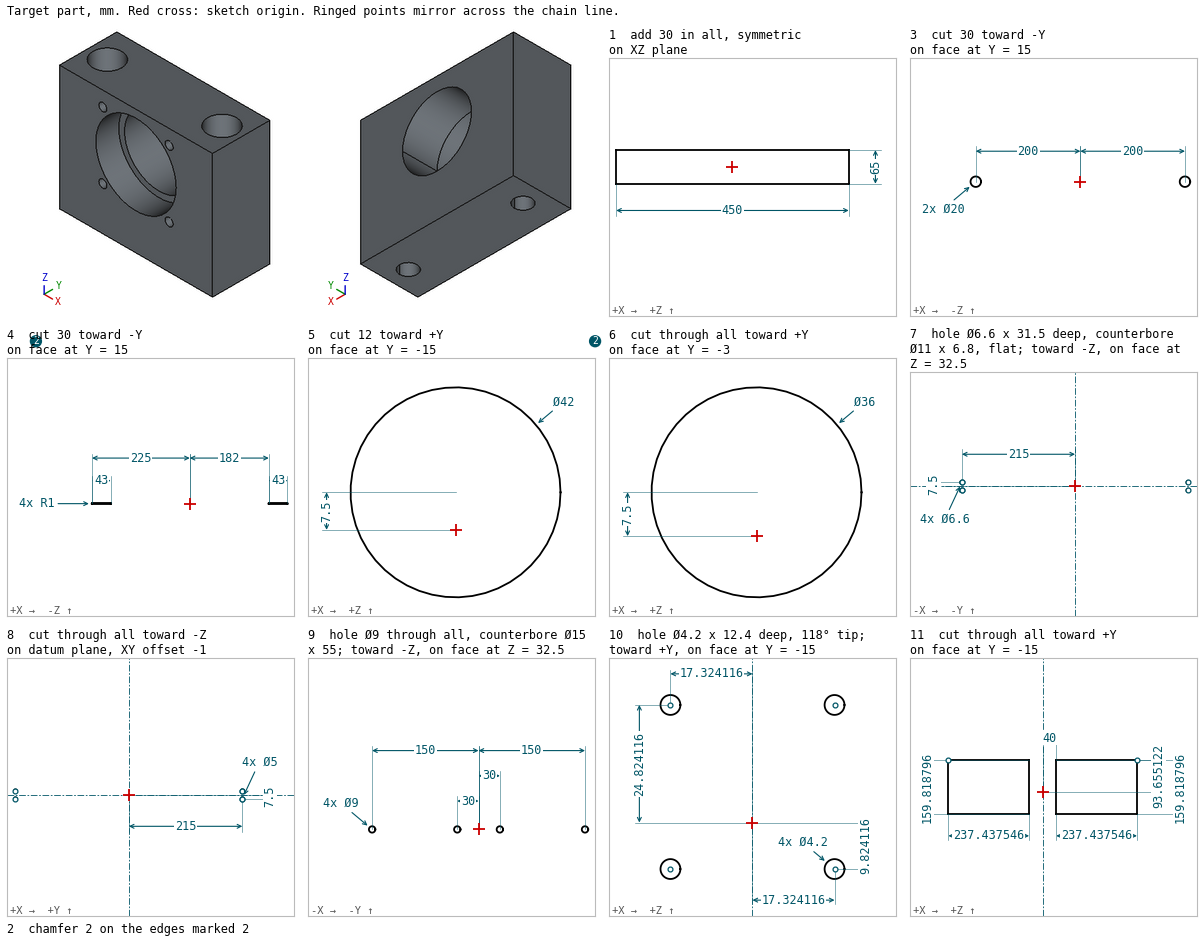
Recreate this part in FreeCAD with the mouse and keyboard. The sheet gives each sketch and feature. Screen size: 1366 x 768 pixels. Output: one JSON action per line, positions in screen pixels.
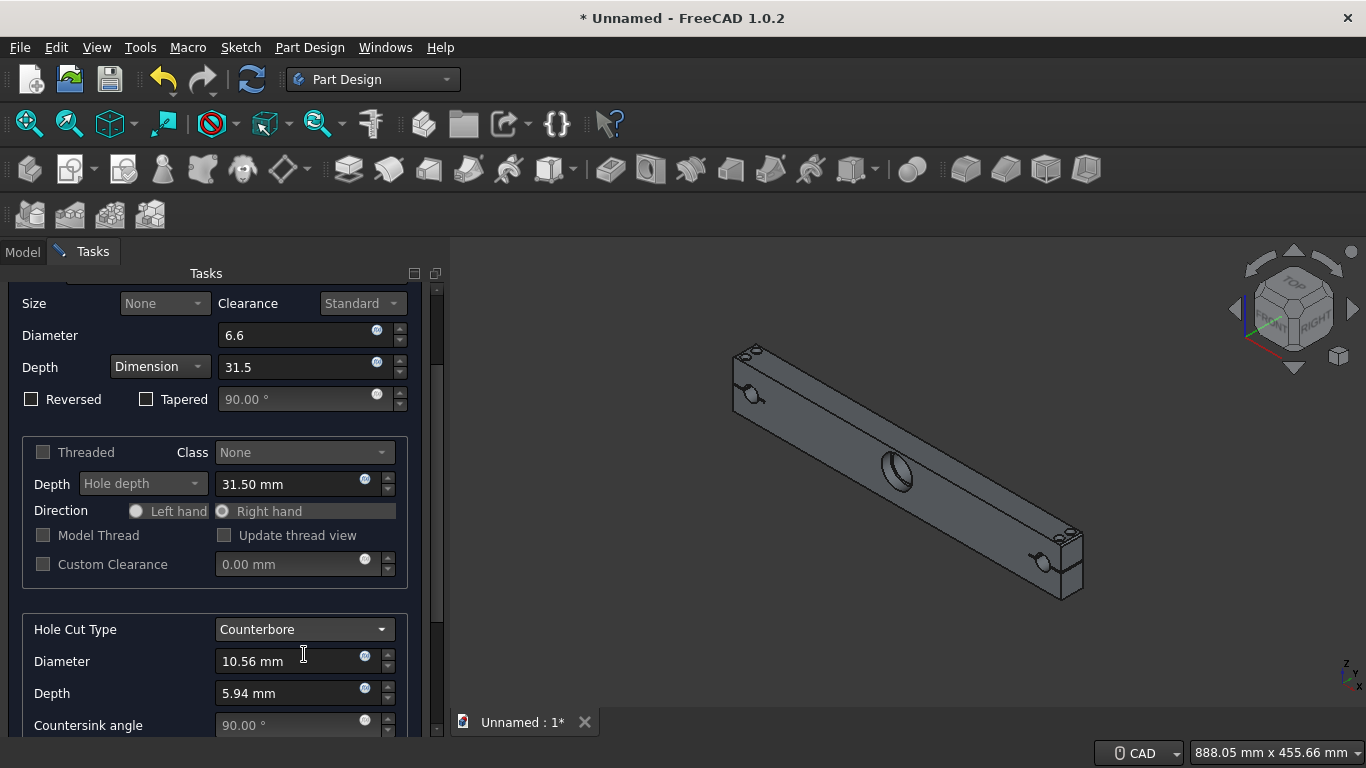
{"action": "triple_click", "coordinate": [298, 661]}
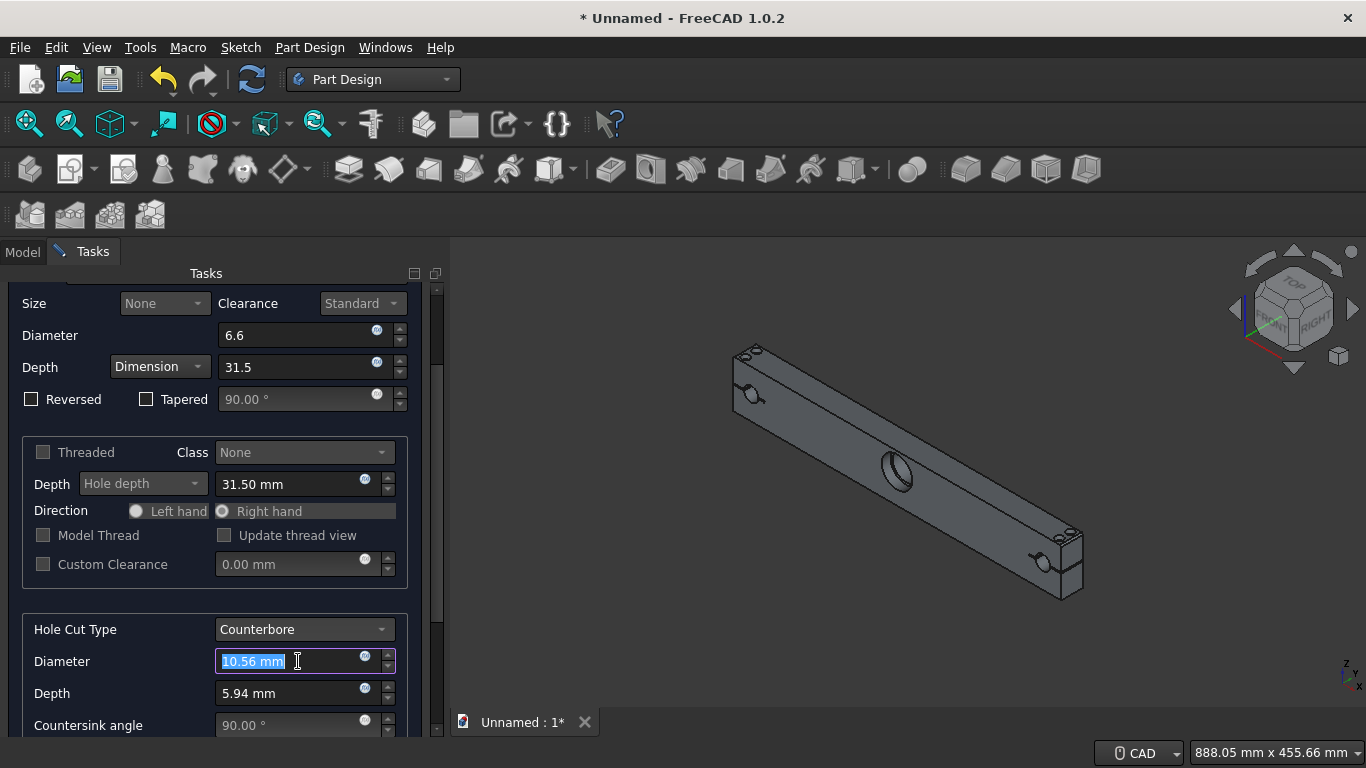
{"action": "type", "text": "11"}
{"action": "key", "text": "Tab"}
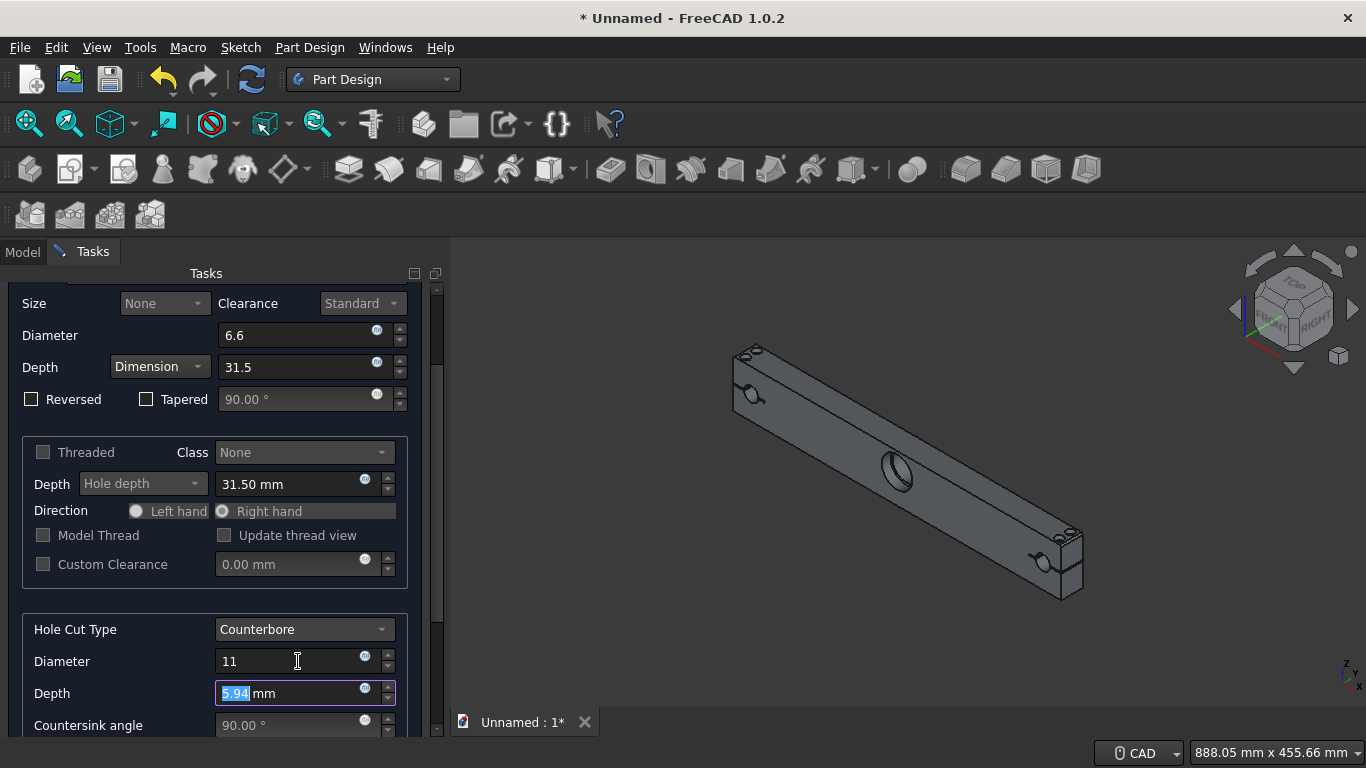
{"action": "type", "text": "6.8"}
{"action": "key", "text": "Tab"}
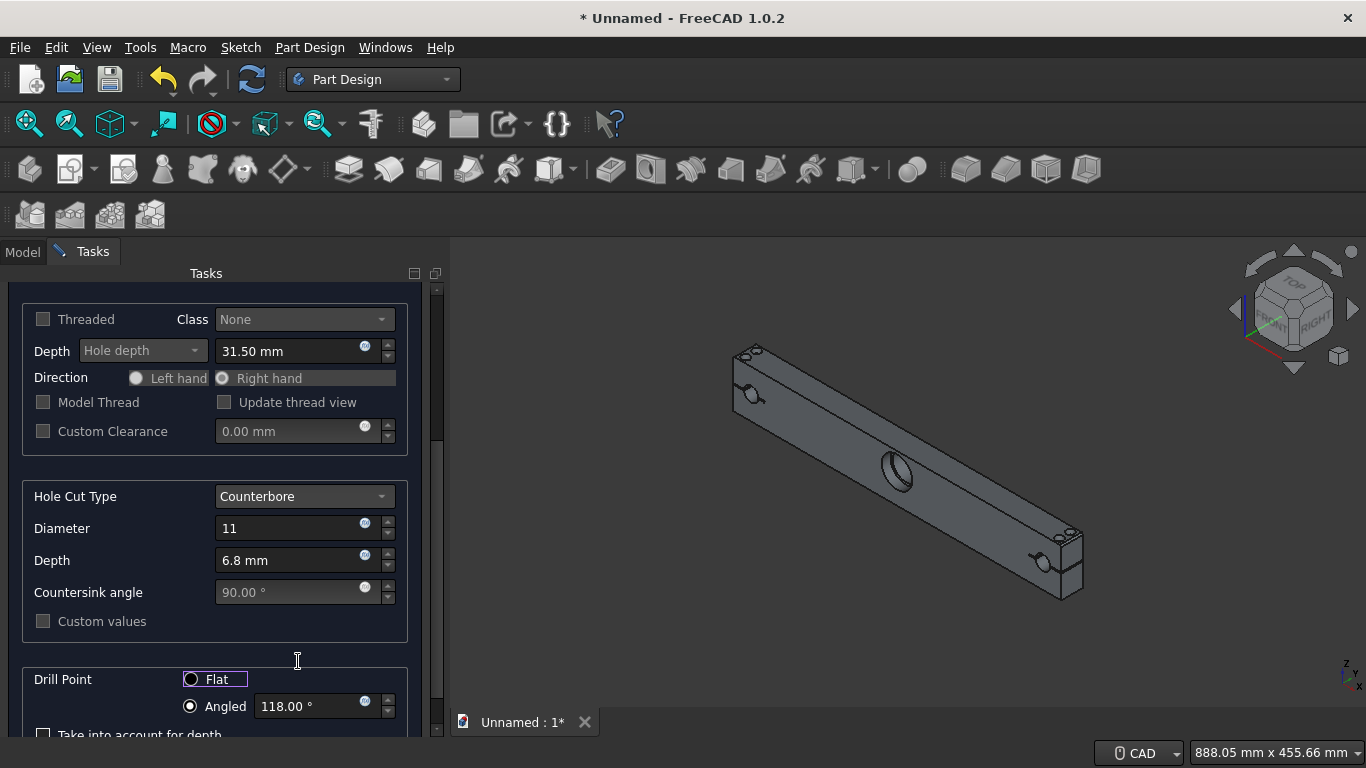
{"action": "left_click", "coordinate": [191, 679]}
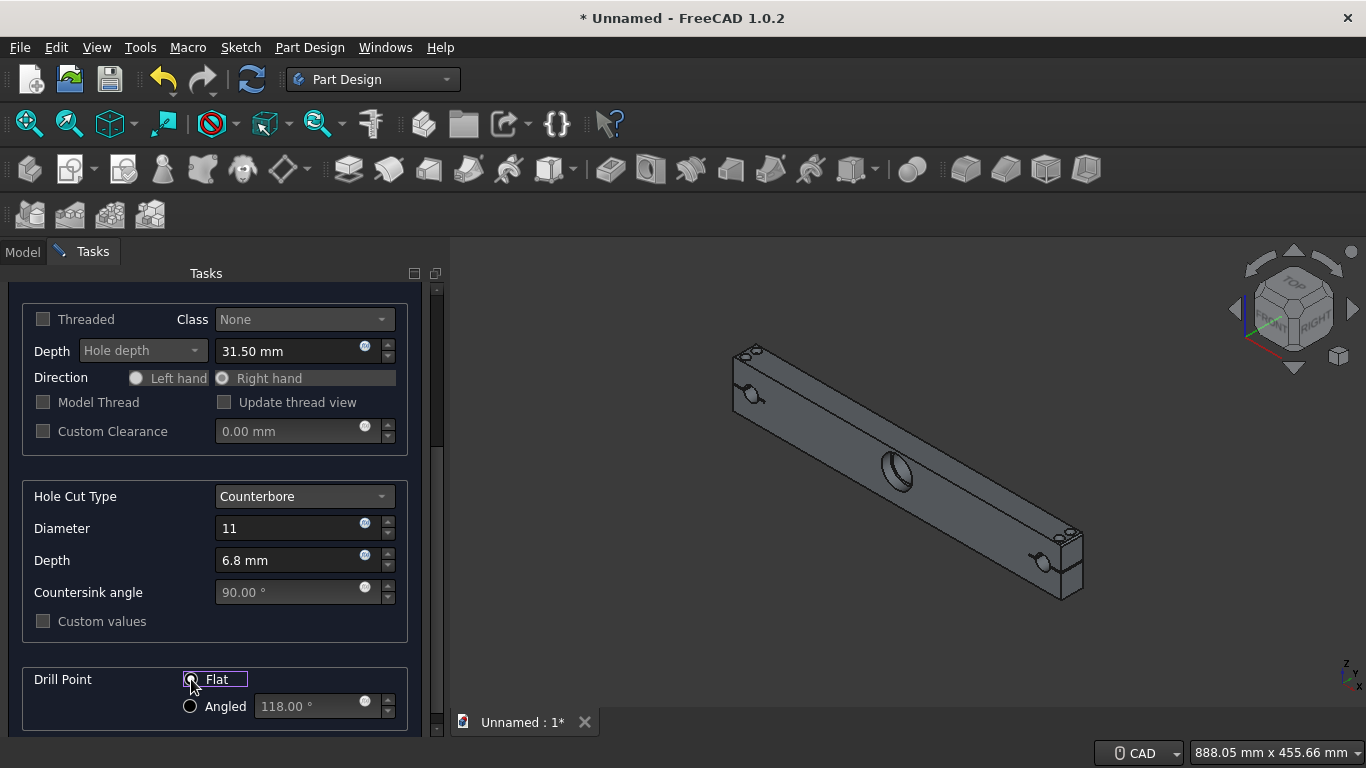
{"action": "scroll", "coordinate": [437, 510], "scroll_direction": "up", "scroll_amount": 5}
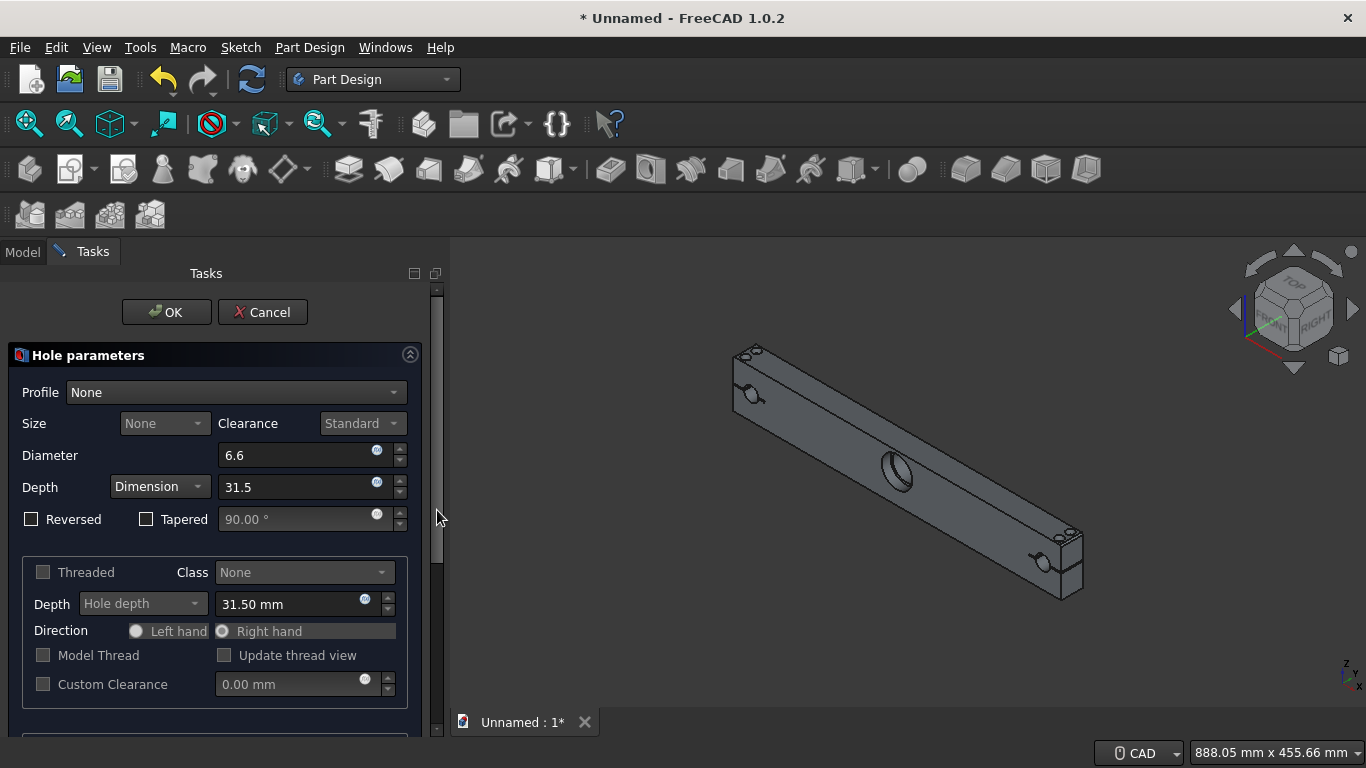
{"action": "left_click", "coordinate": [167, 312]}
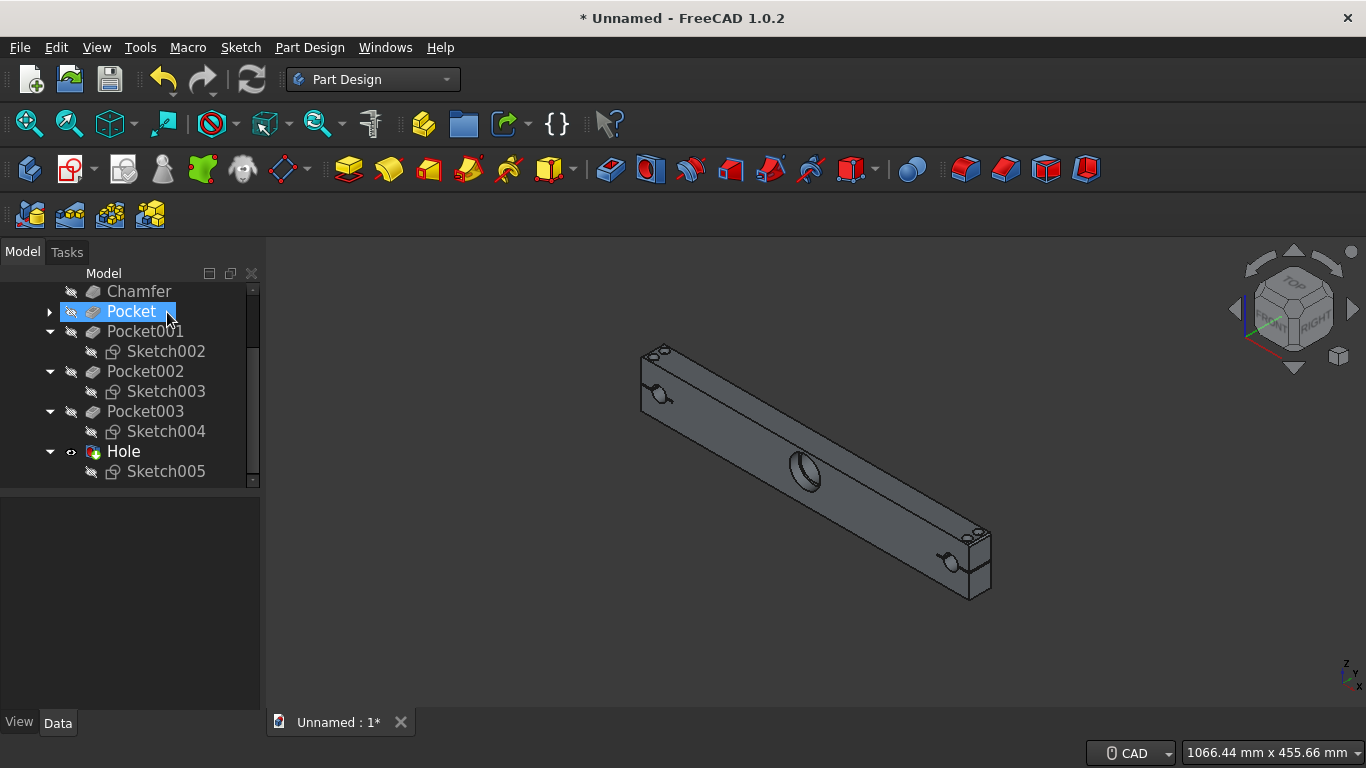
{"action": "key", "text": "2"}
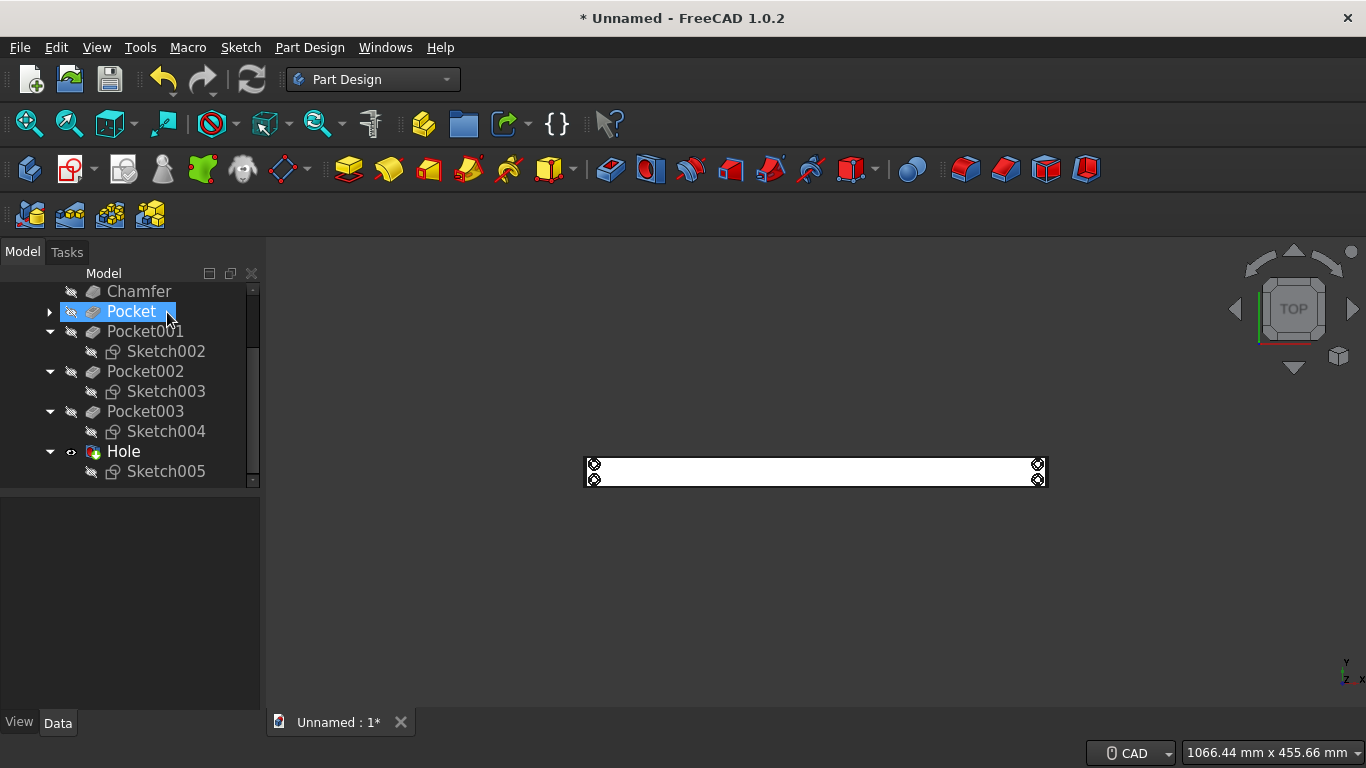
{"action": "key", "text": "v f"}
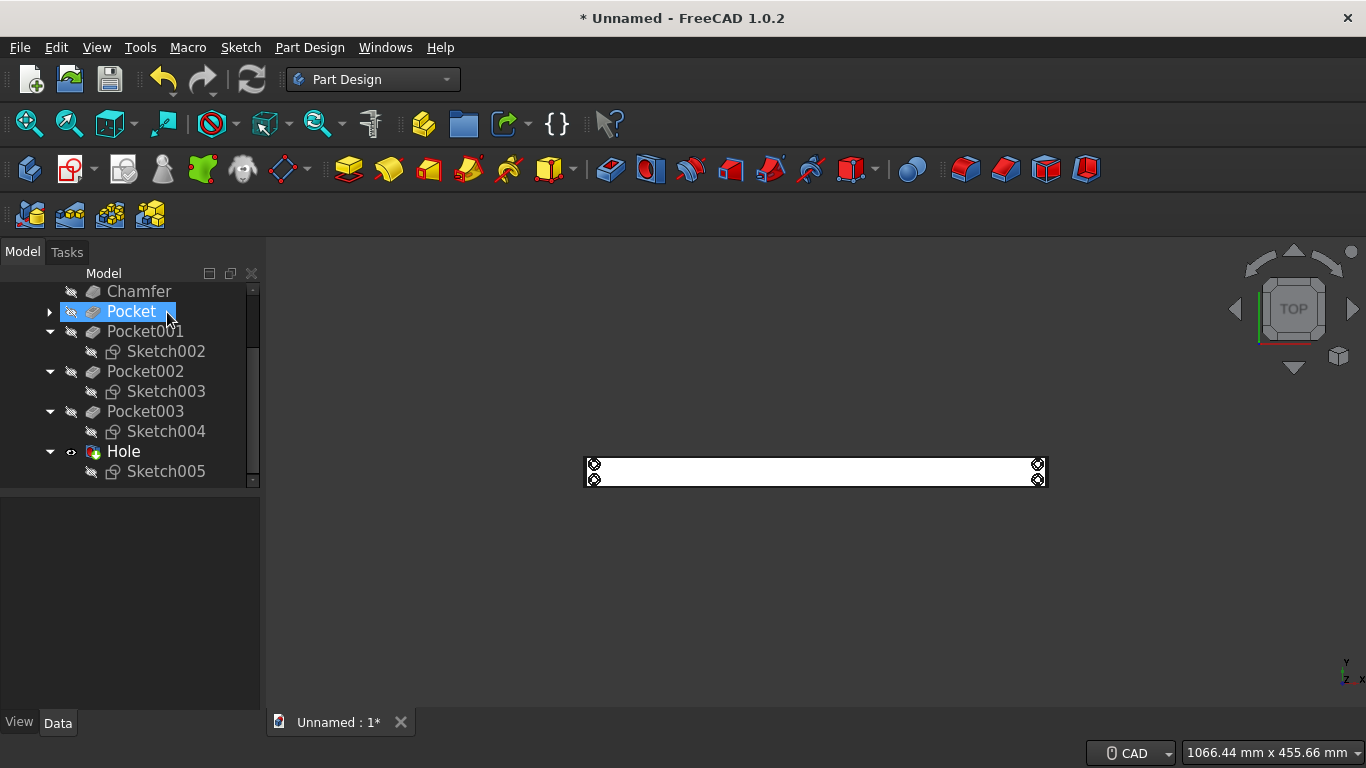
{"action": "key", "text": "0"}